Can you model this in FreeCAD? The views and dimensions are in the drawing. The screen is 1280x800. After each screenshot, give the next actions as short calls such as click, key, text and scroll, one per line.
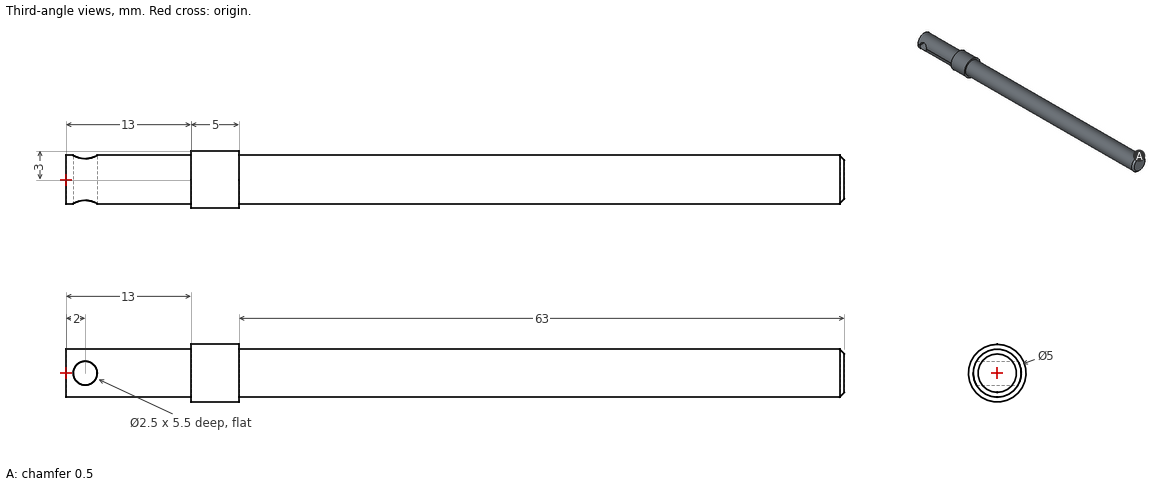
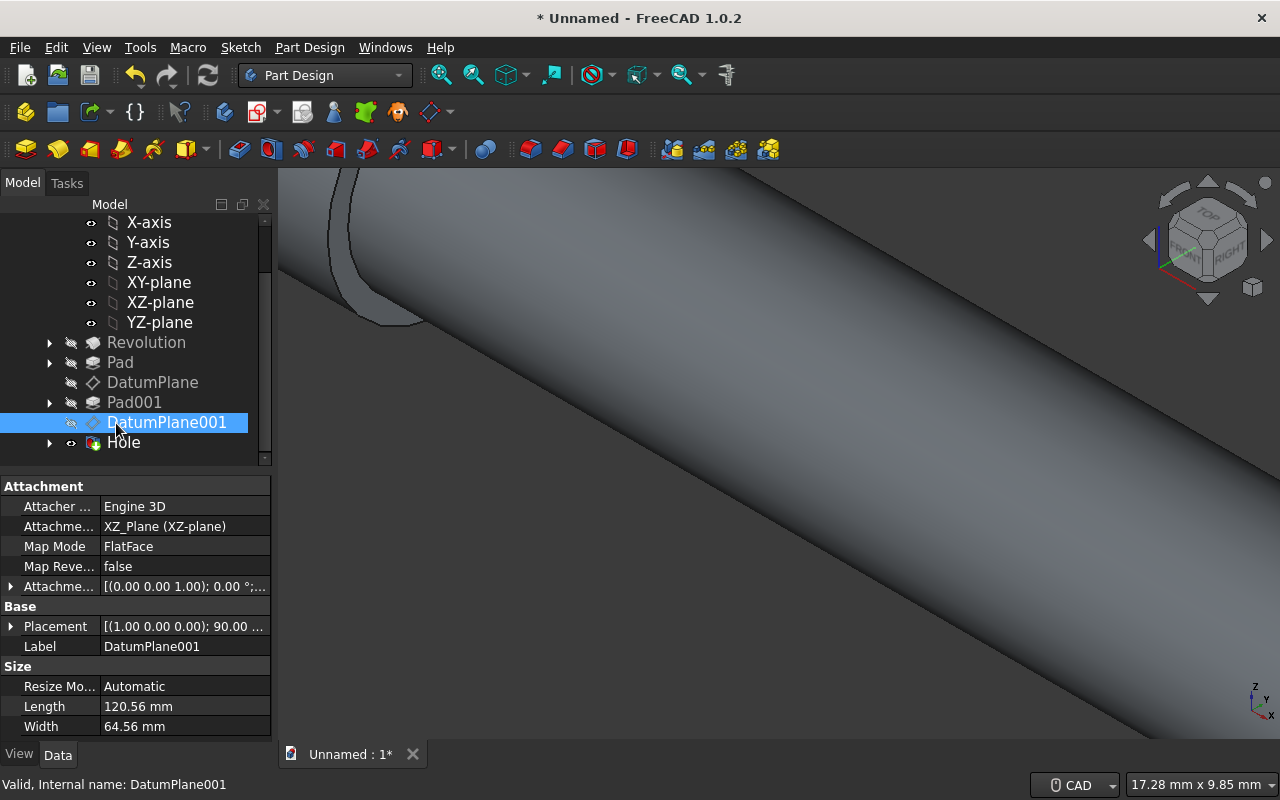
click(442, 76)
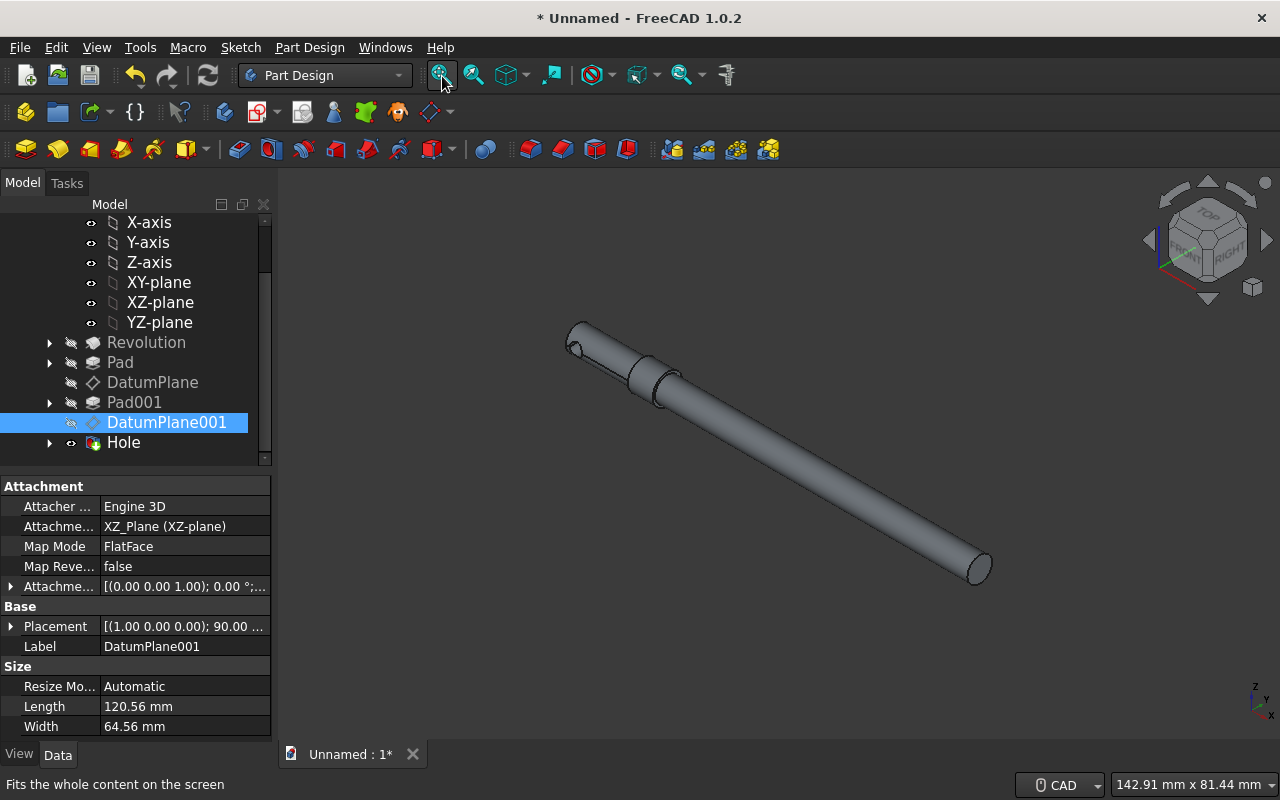
click(967, 576)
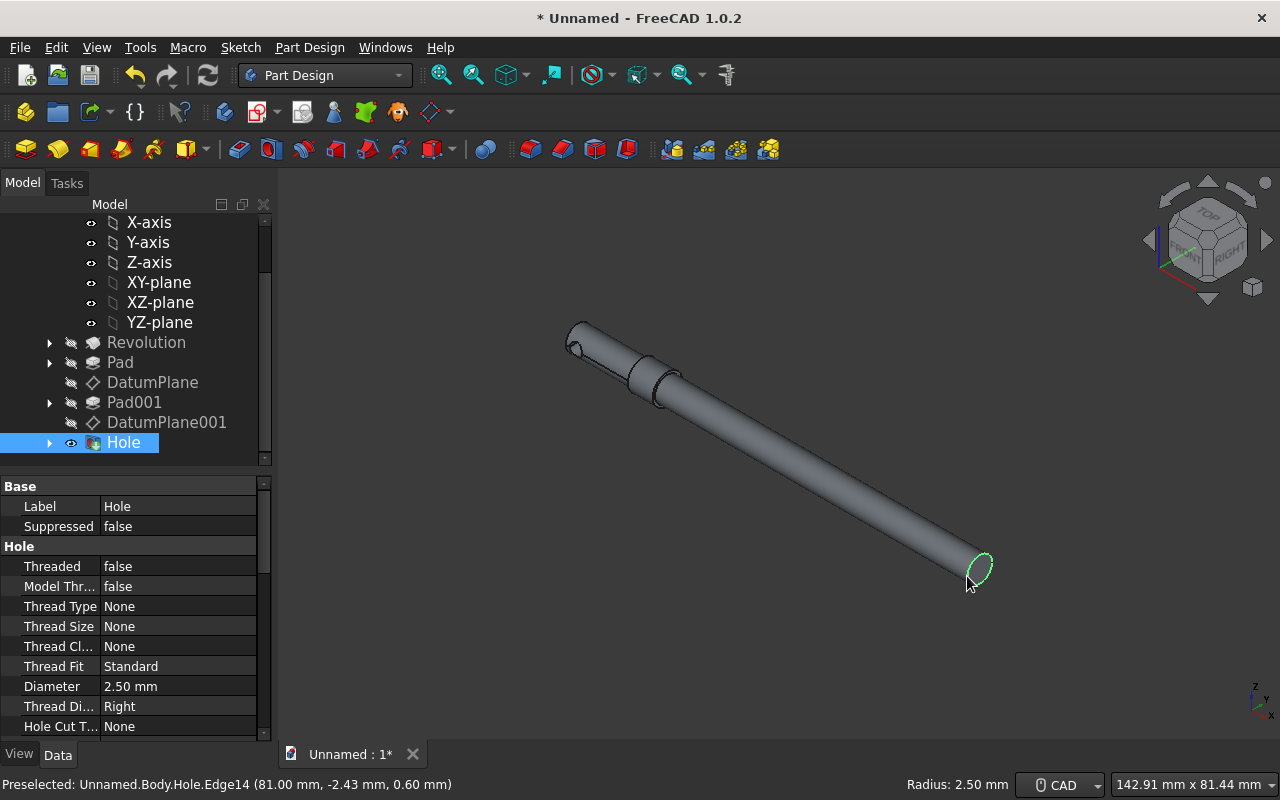
click(564, 150)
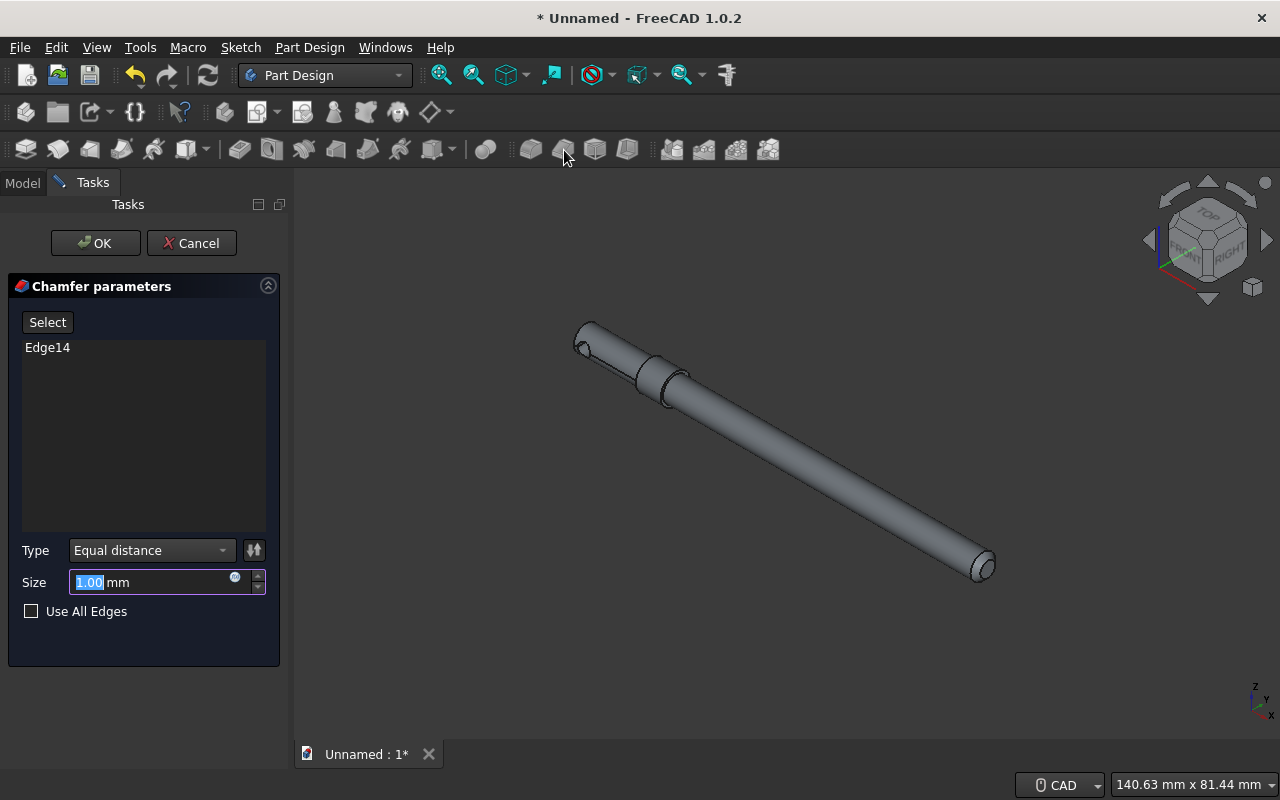
text(0.5)
key(Tab)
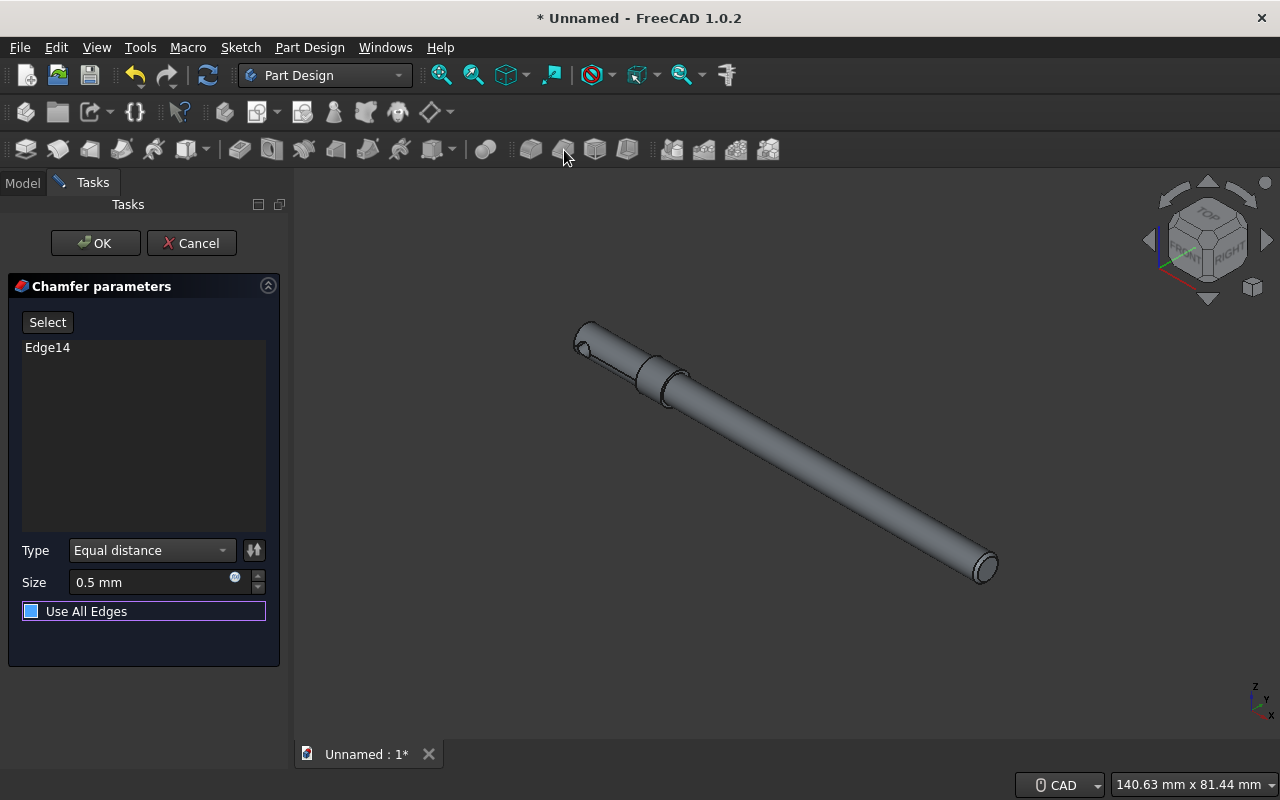
click(96, 243)